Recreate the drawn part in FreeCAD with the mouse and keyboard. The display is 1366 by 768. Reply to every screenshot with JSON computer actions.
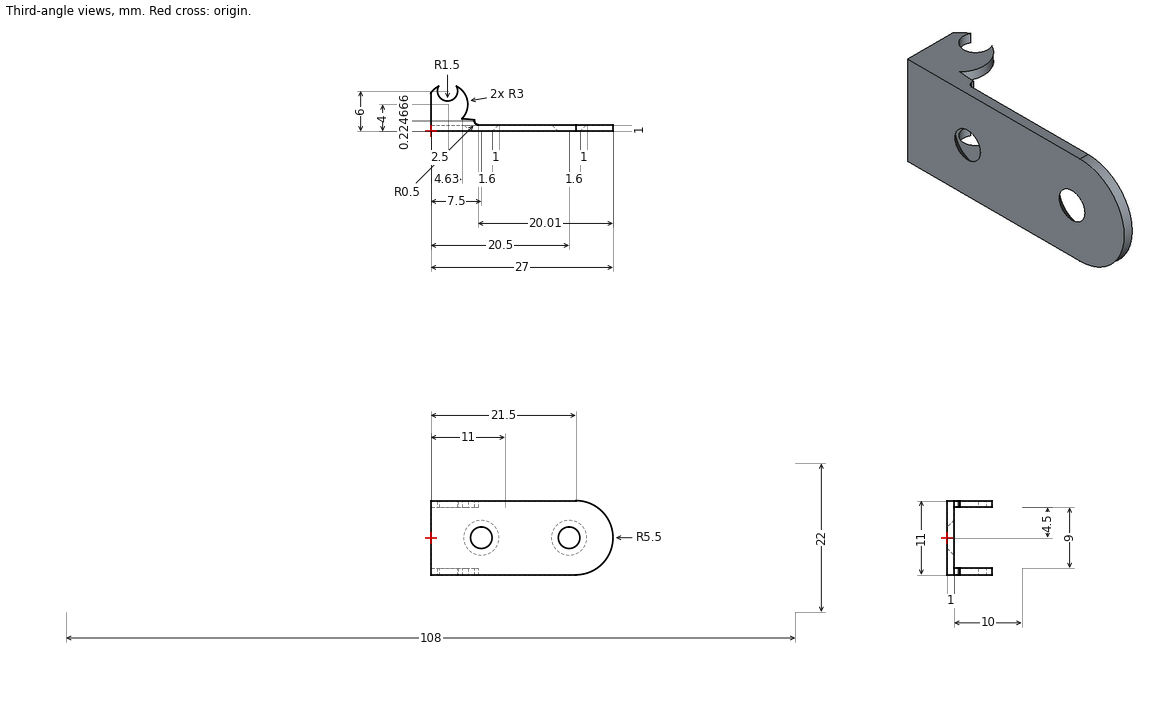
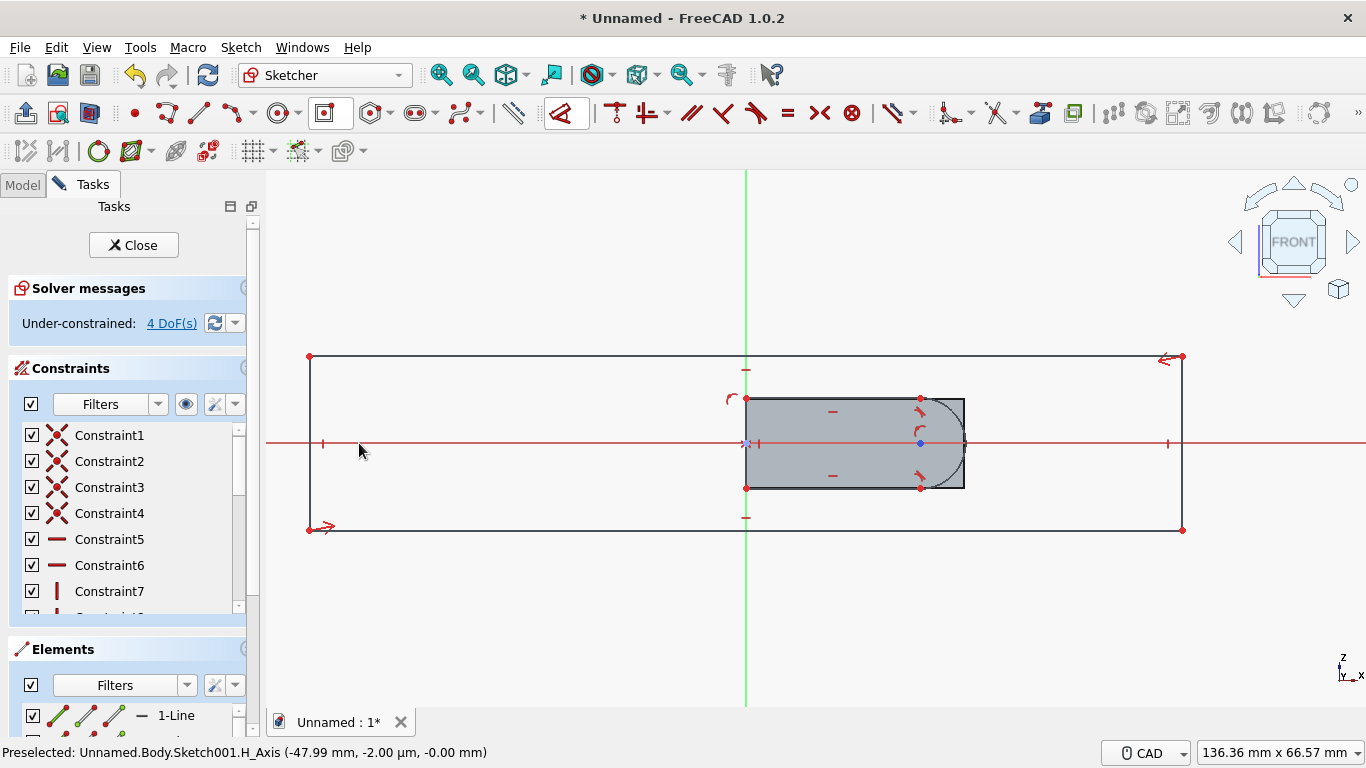
{"action": "left_click", "coordinate": [560, 114]}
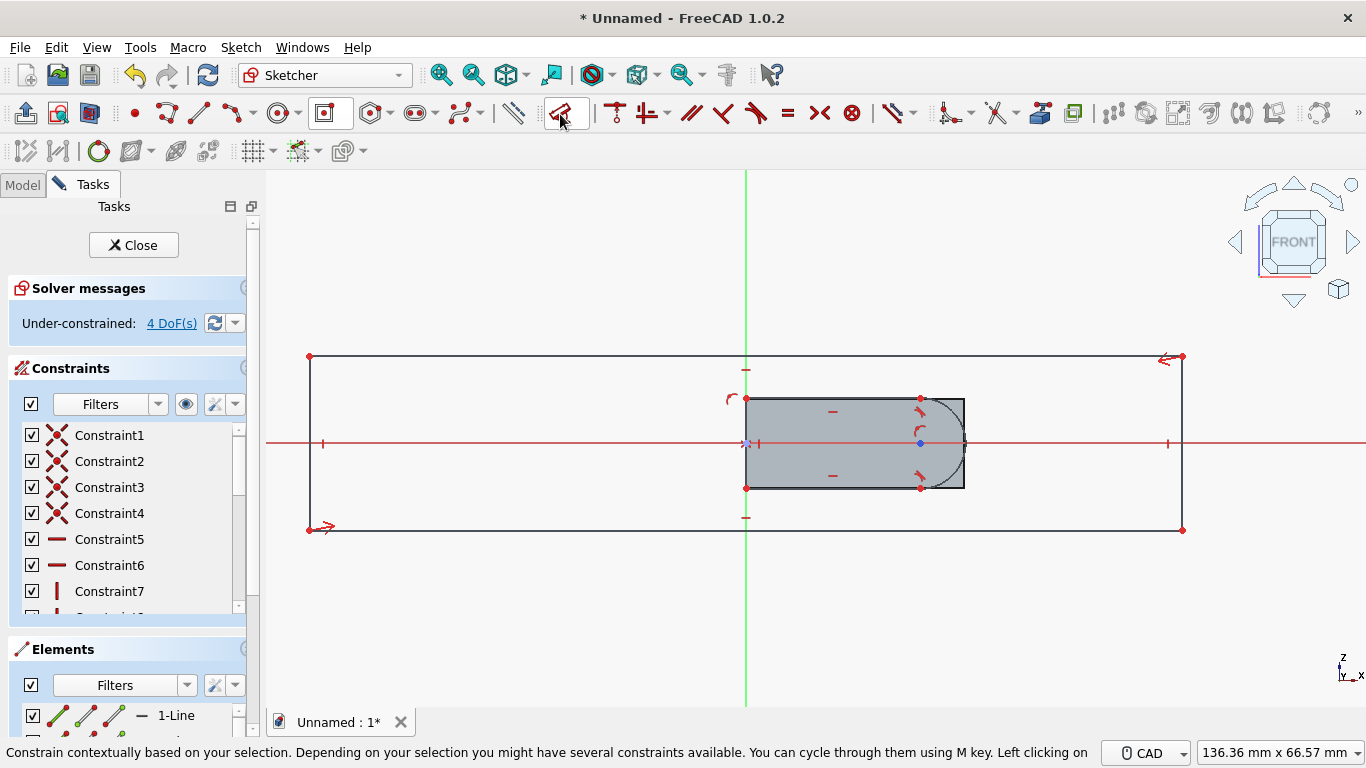
{"action": "left_click", "coordinate": [957, 470]}
{"action": "left_click", "coordinate": [983, 489]}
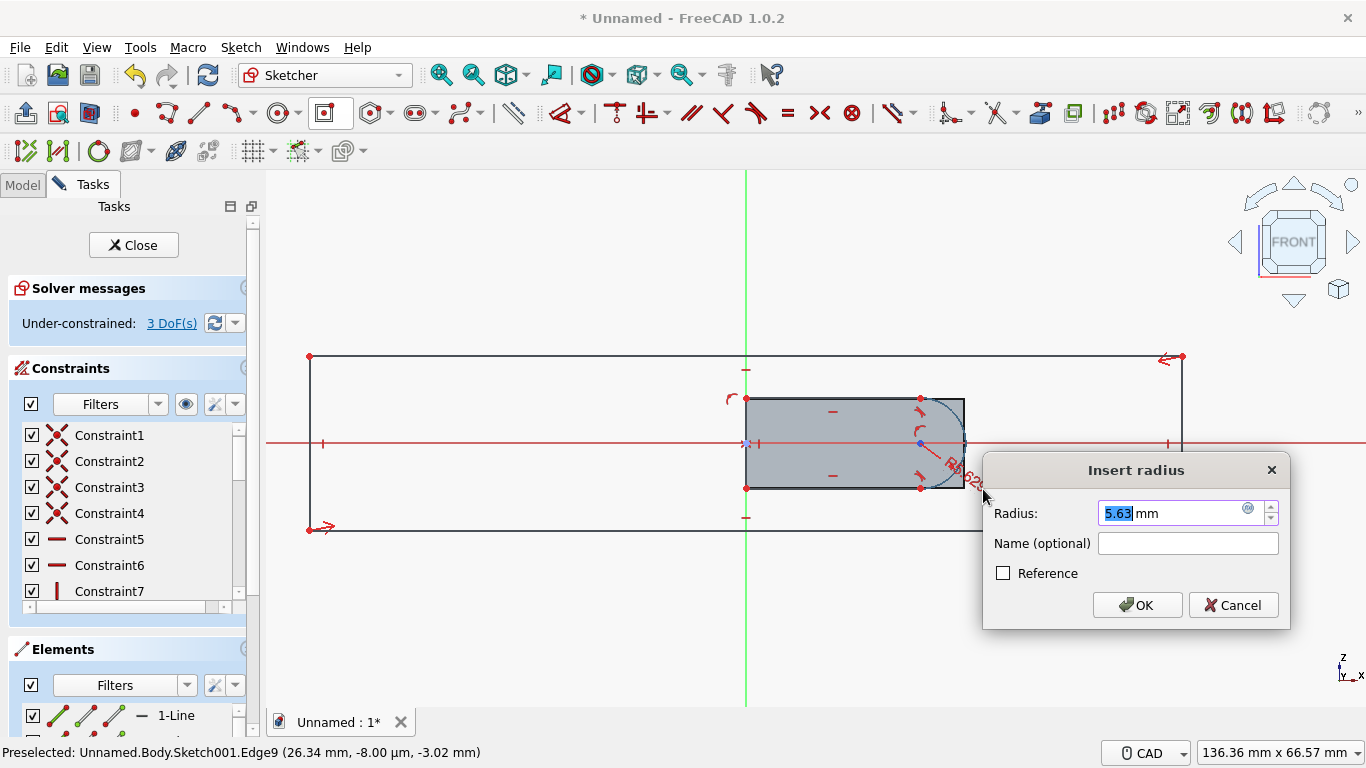
{"action": "type", "text": "5.5"}
{"action": "key", "text": "Return"}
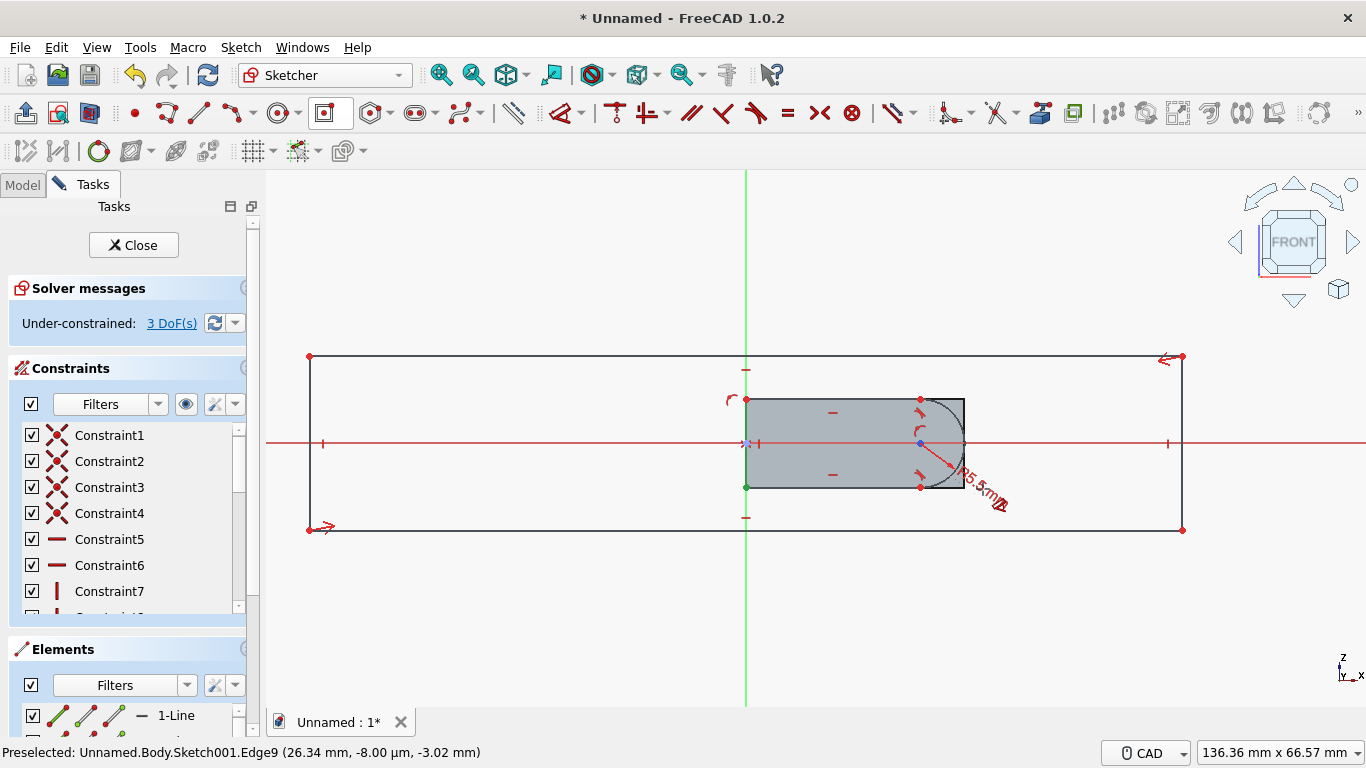
{"action": "left_click", "coordinate": [1182, 478]}
{"action": "left_click", "coordinate": [1148, 403]}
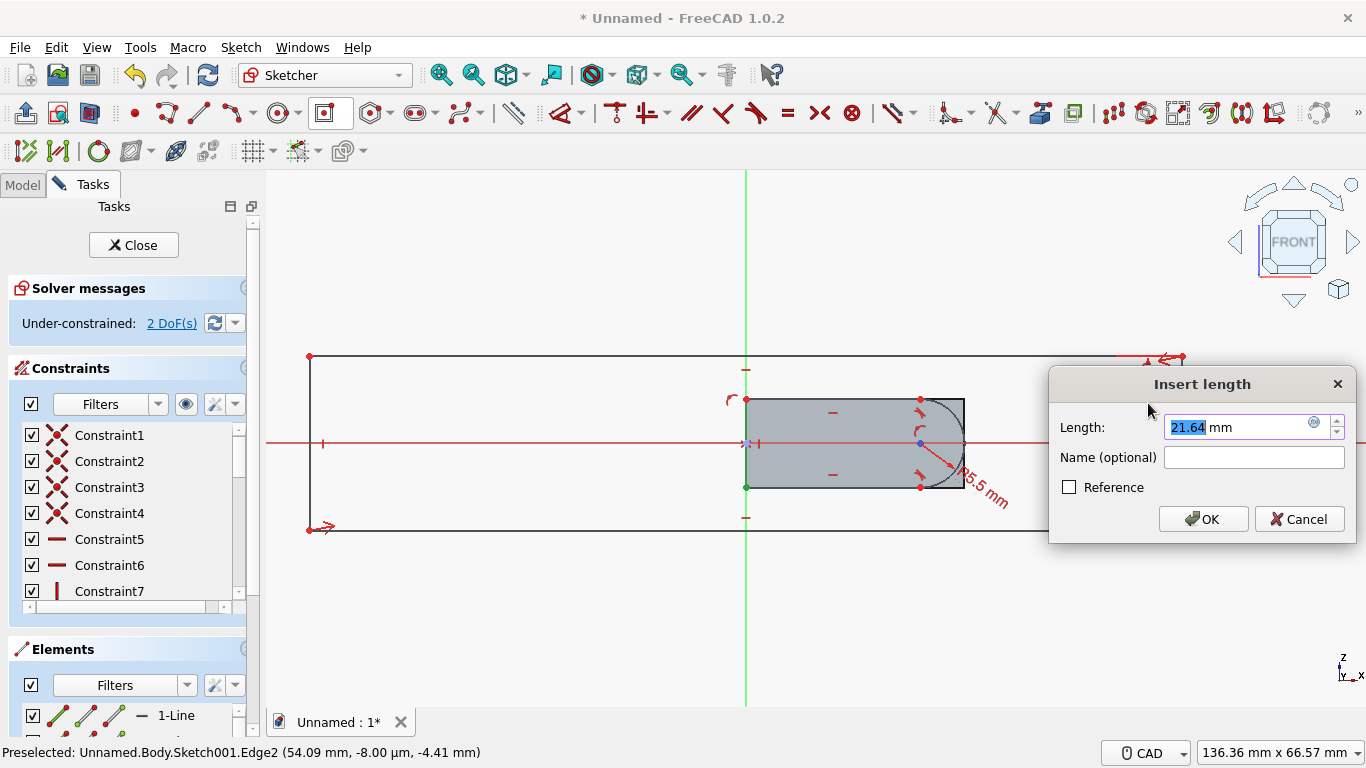
{"action": "type", "text": "22"}
{"action": "key", "text": "Return"}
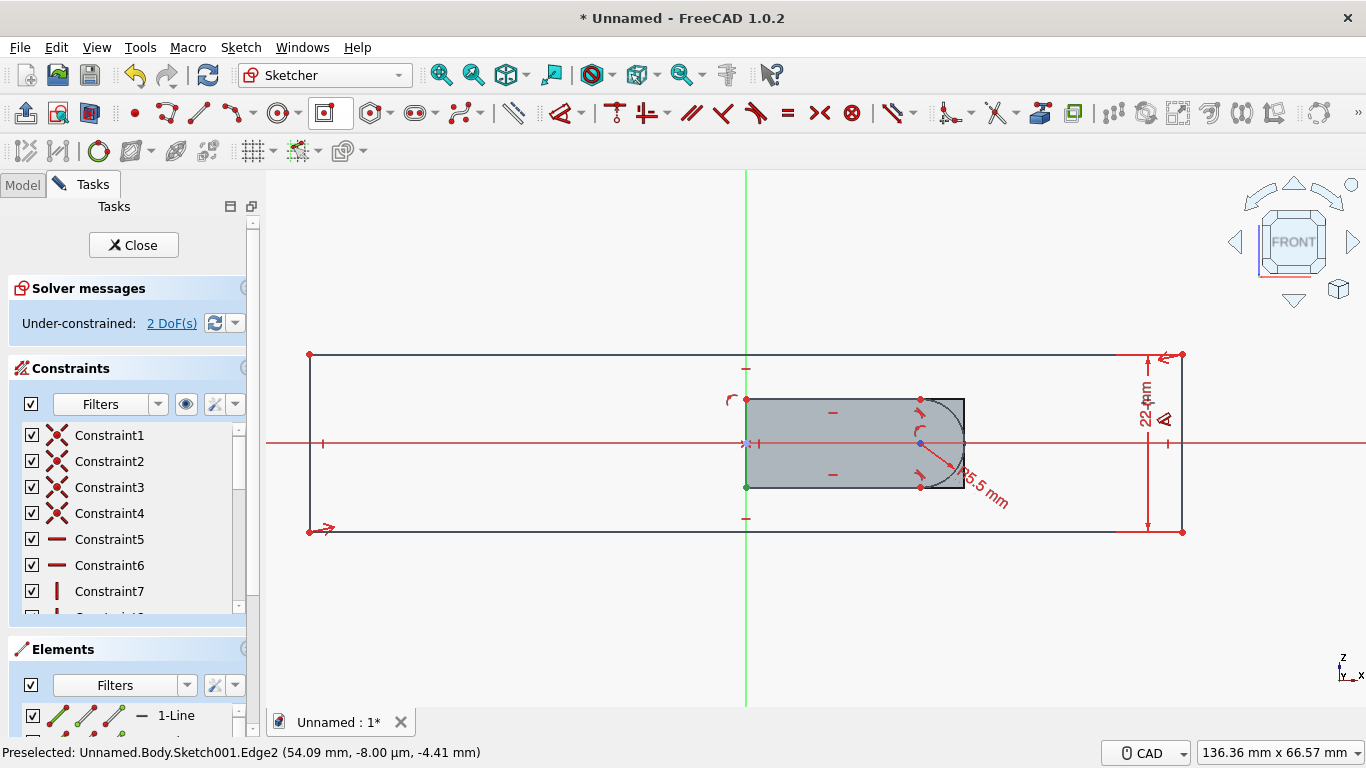
{"action": "left_click", "coordinate": [572, 532]}
{"action": "left_click", "coordinate": [545, 566]}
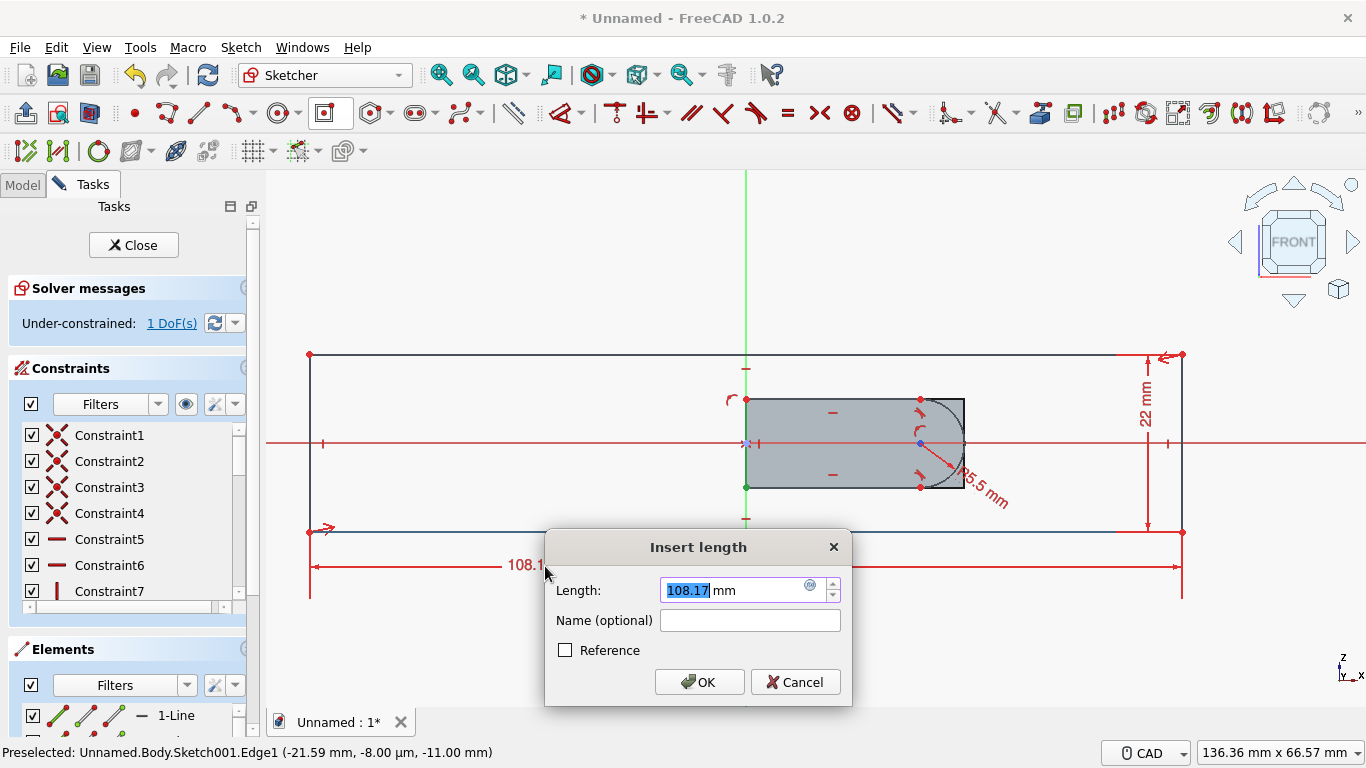
{"action": "type", "text": "108"}
{"action": "key", "text": "Return"}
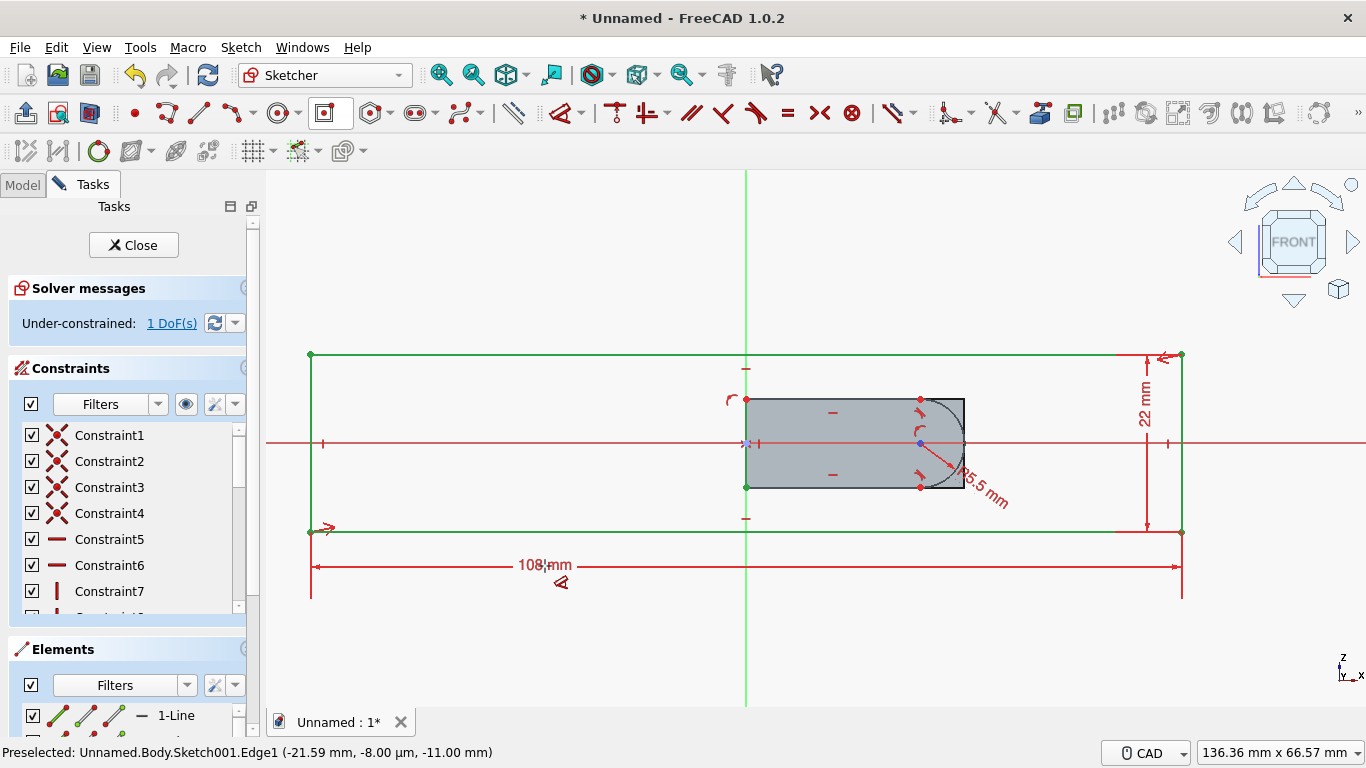
{"action": "left_click", "coordinate": [868, 399]}
{"action": "left_click", "coordinate": [833, 341]}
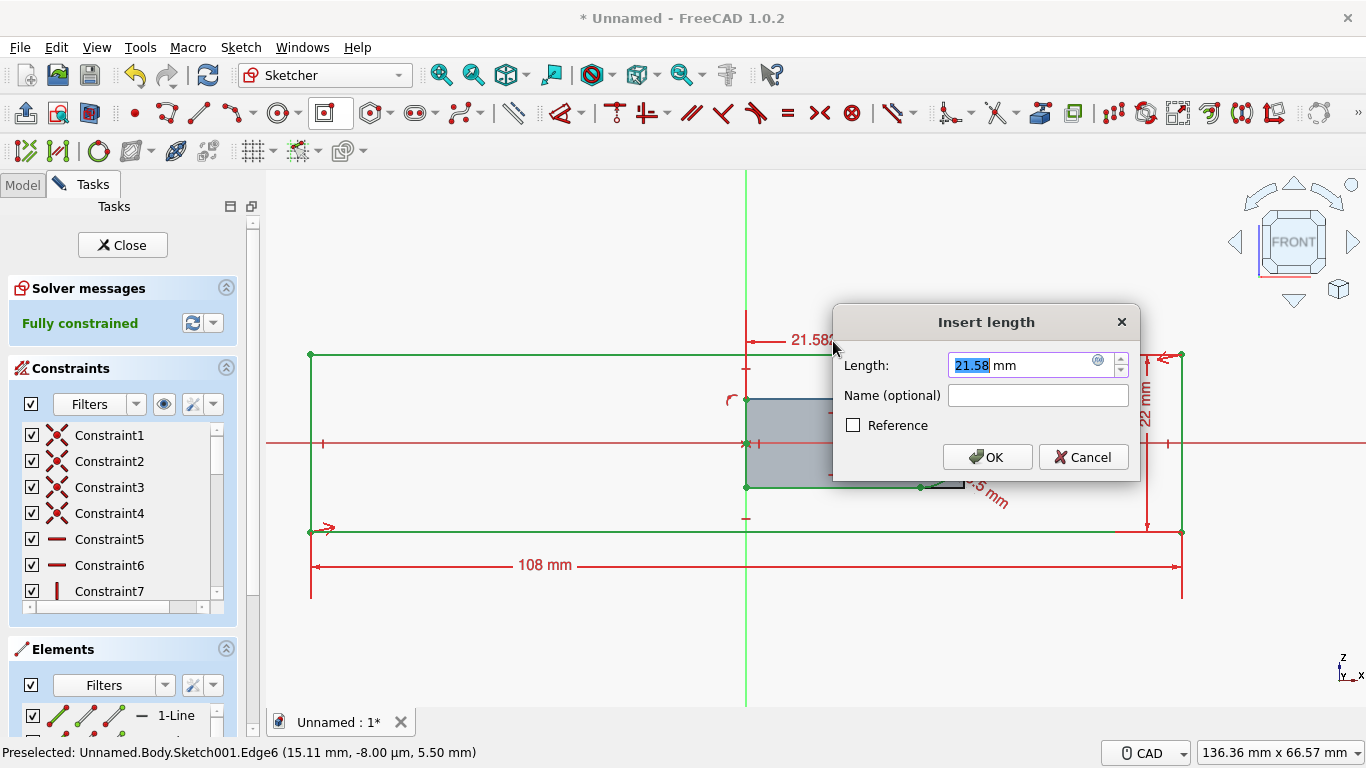
{"action": "type", "text": "21.5"}
{"action": "key", "text": "Return"}
{"action": "key", "text": "Escape"}